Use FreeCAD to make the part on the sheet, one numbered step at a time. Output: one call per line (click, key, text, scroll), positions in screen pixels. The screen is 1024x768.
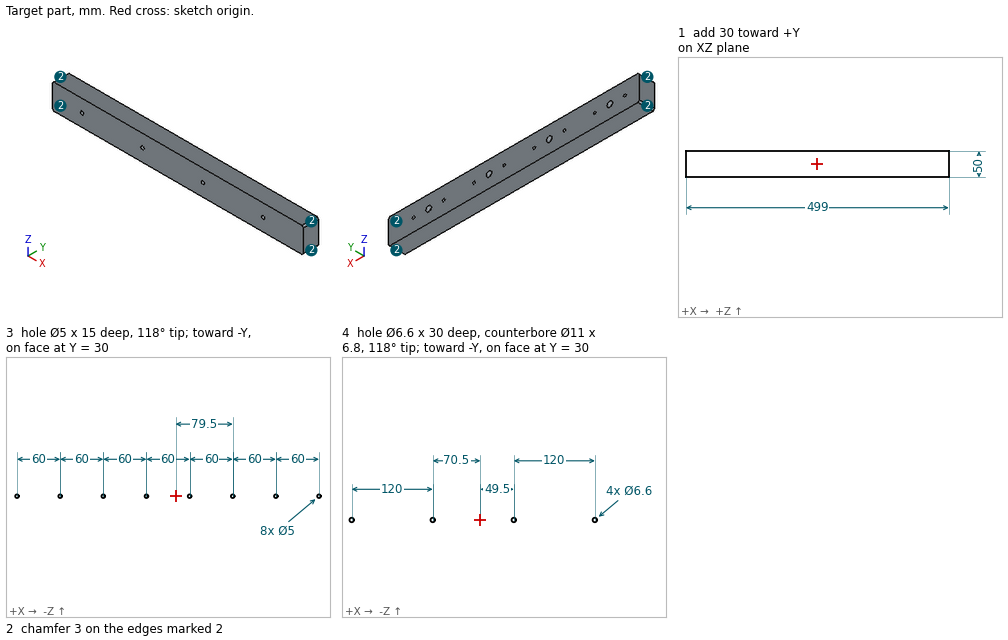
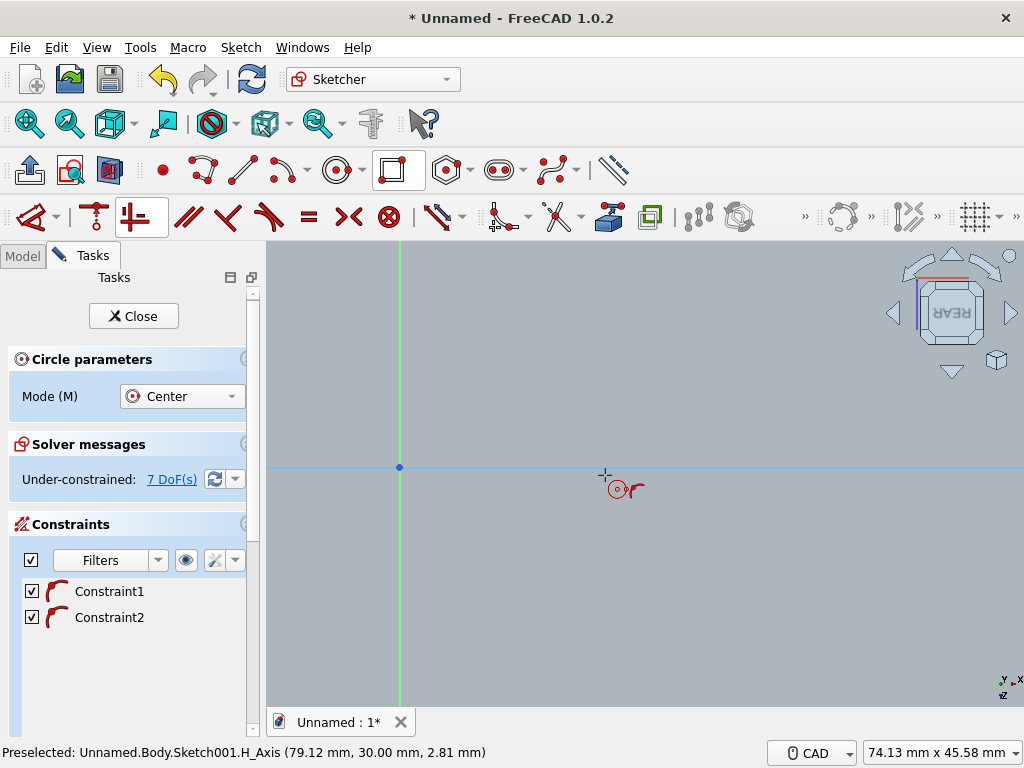
scroll(605, 475, down, 12)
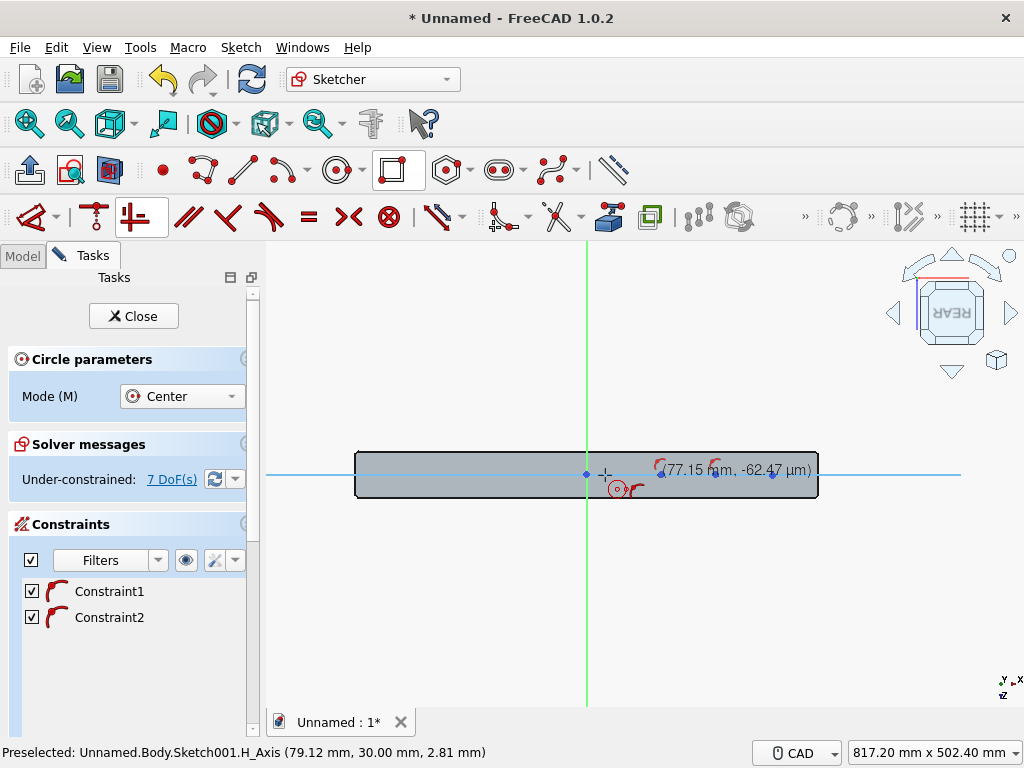
click(605, 475)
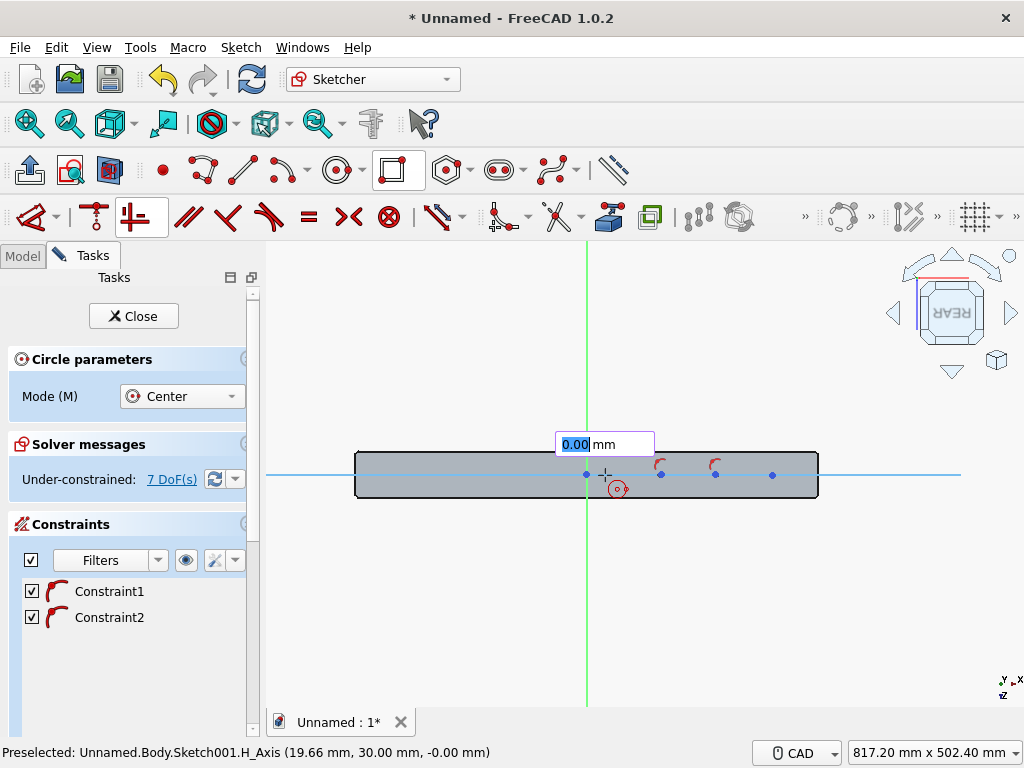
scroll(604, 477, up, 10)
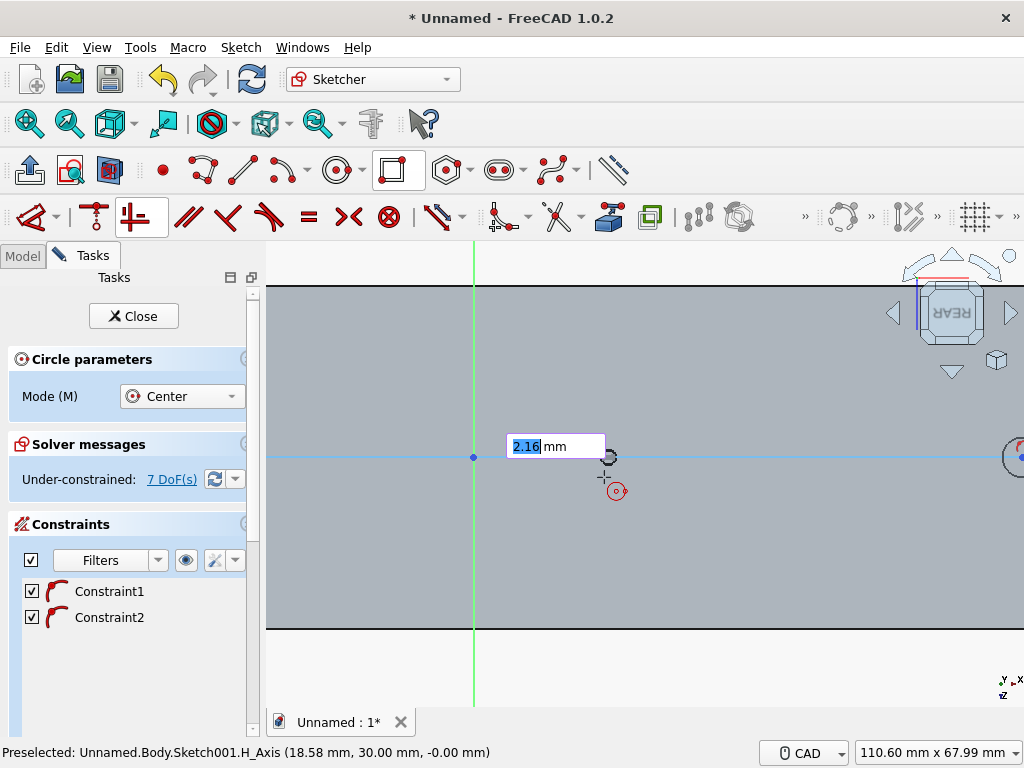
click(602, 474)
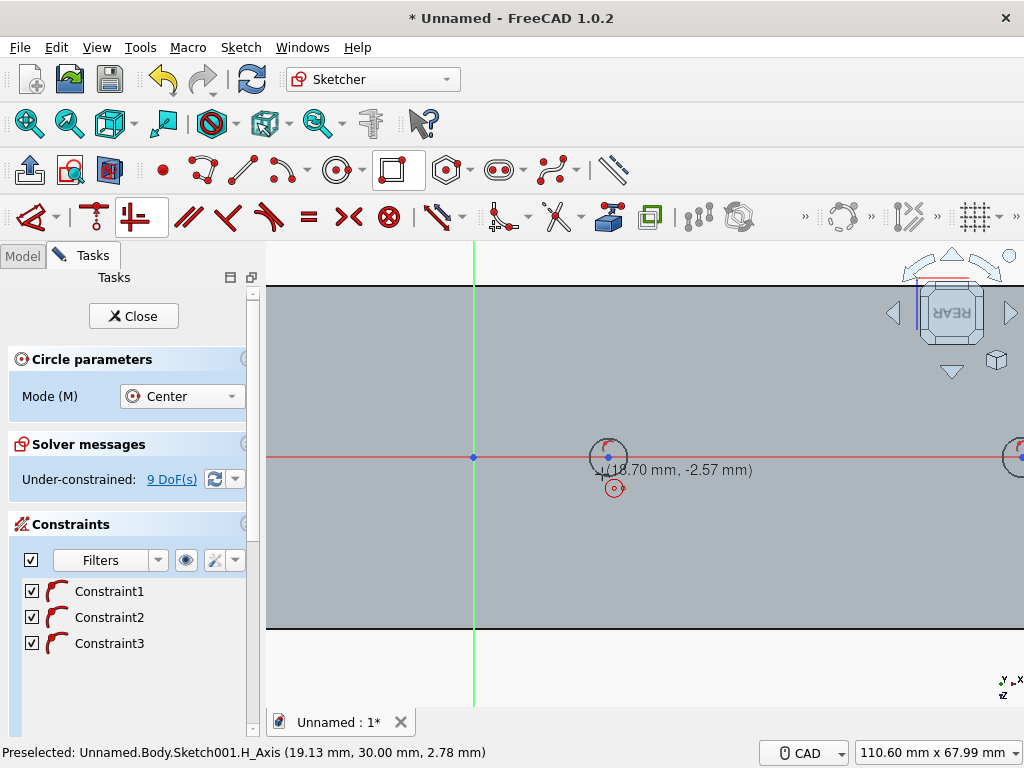
scroll(604, 477, down, 10)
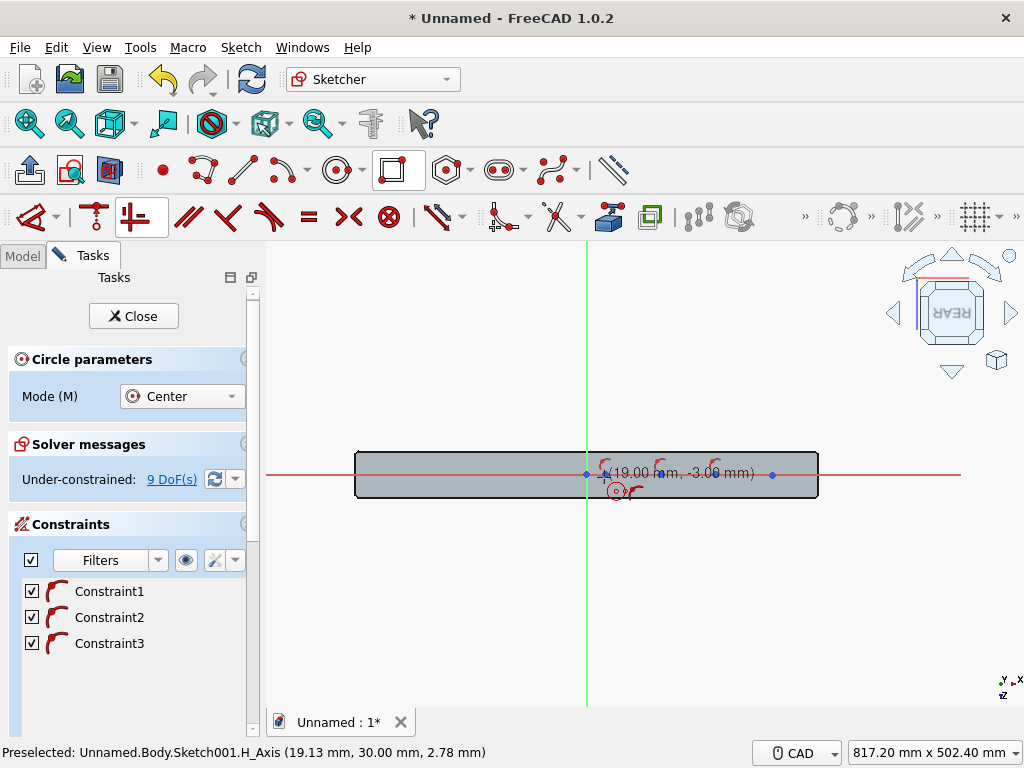
scroll(549, 475, up, 12)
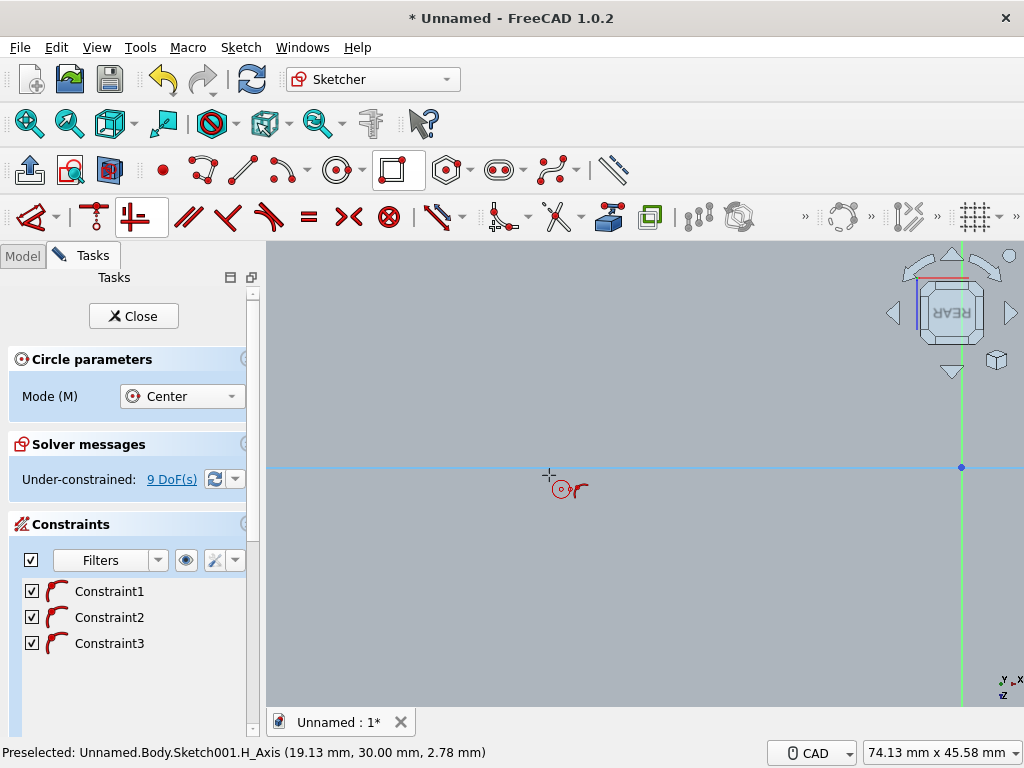
scroll(549, 475, down, 12)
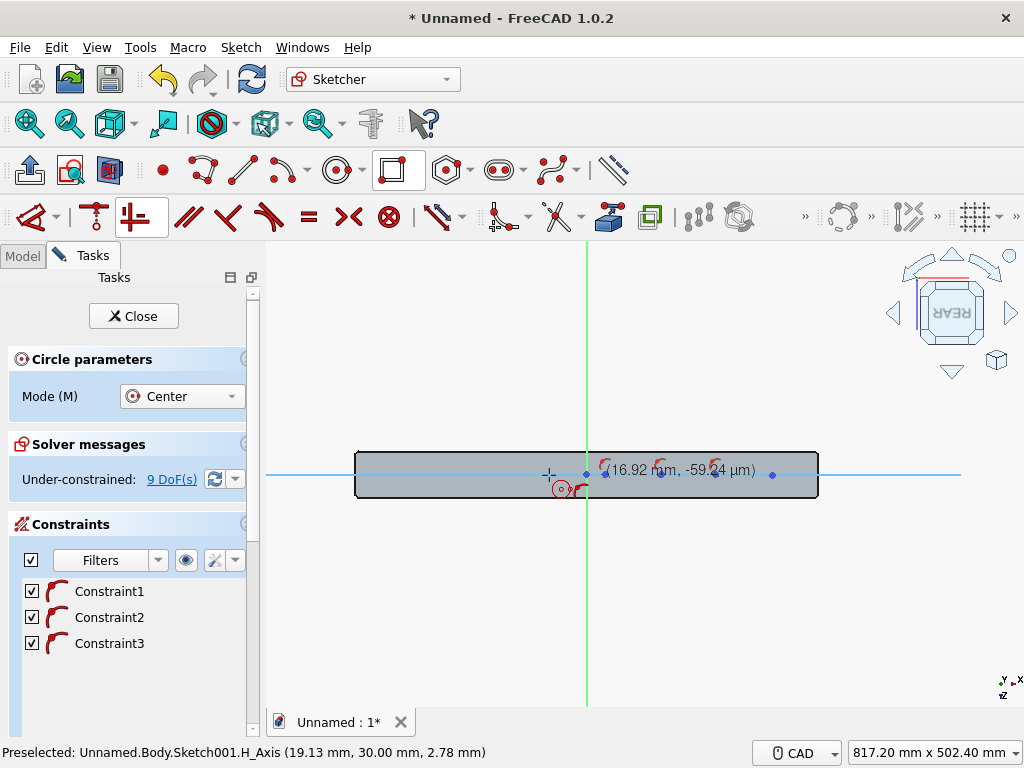
click(549, 475)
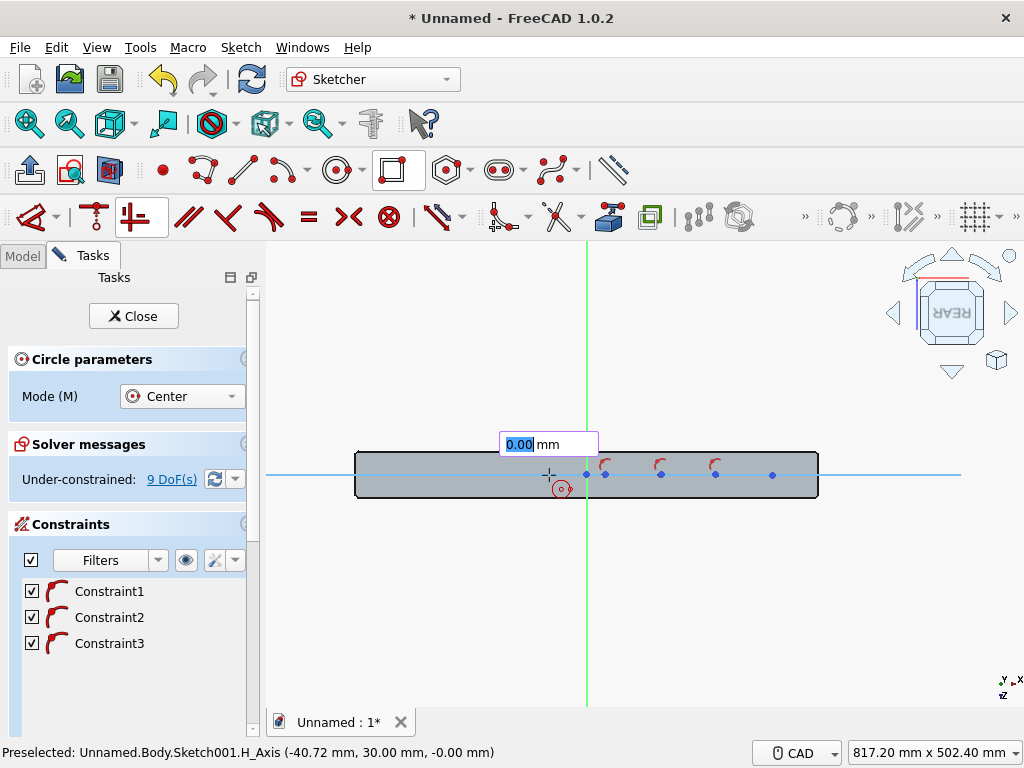
scroll(548, 477, up, 10)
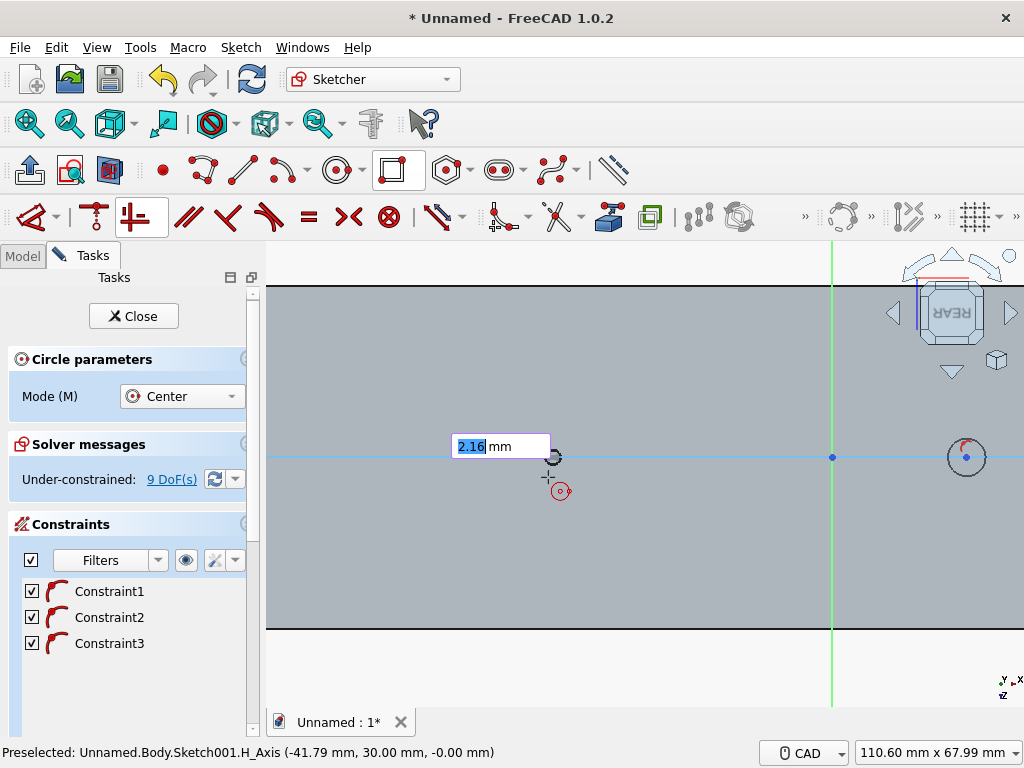
click(549, 474)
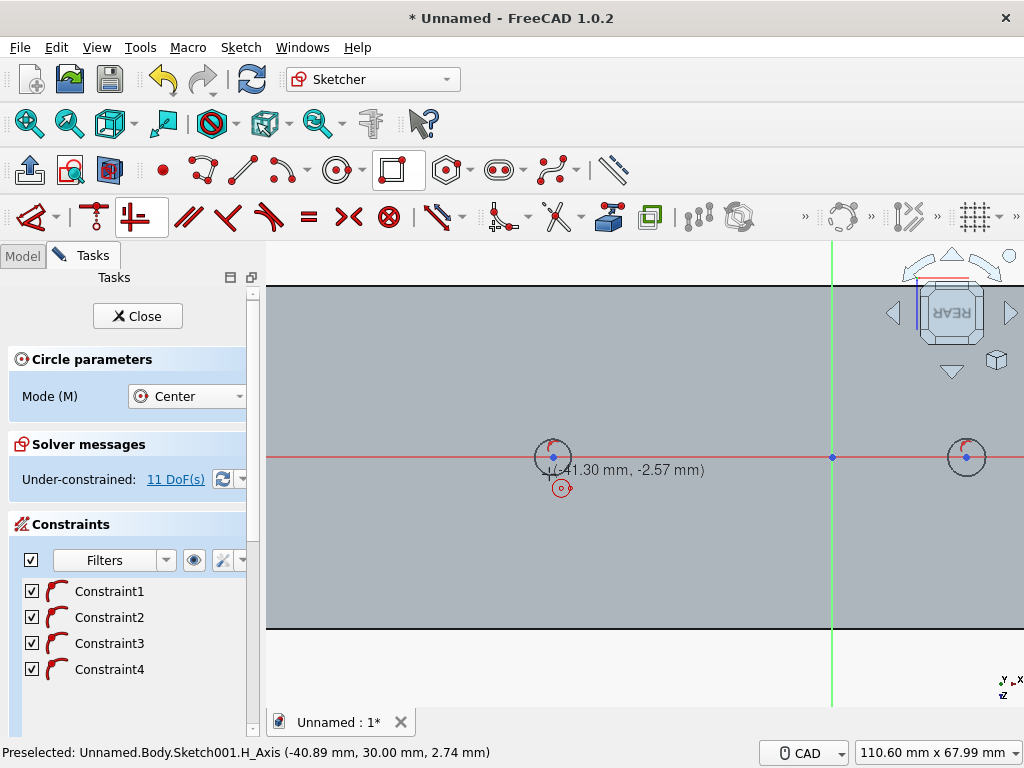
scroll(548, 477, down, 10)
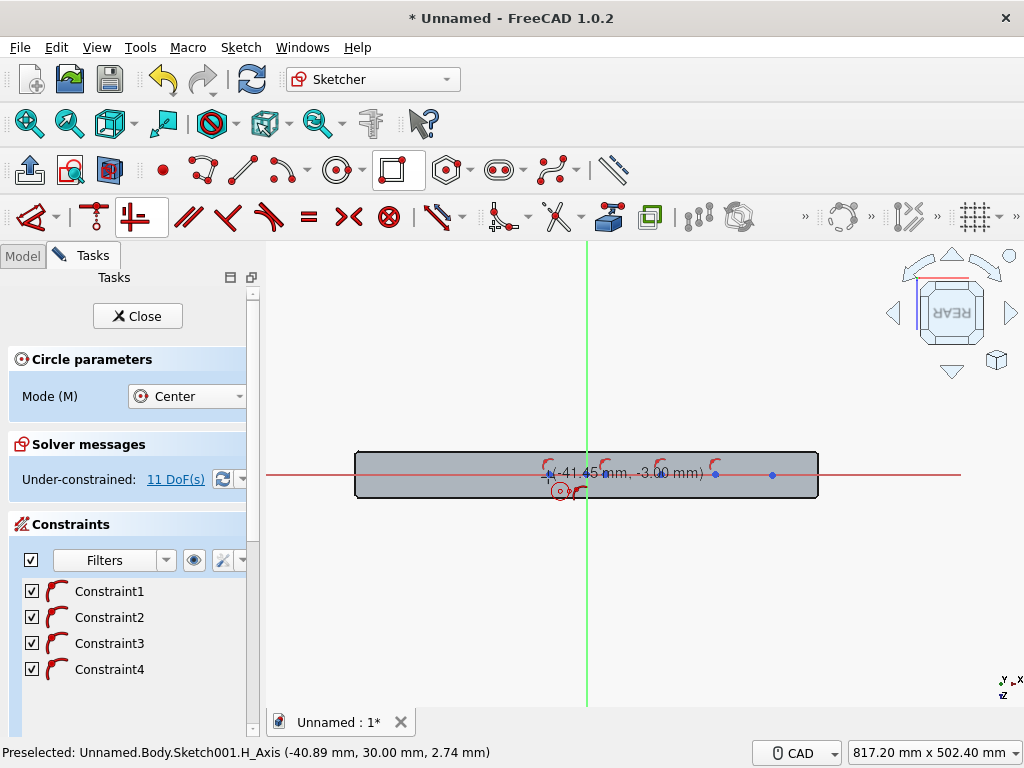
scroll(494, 475, up, 12)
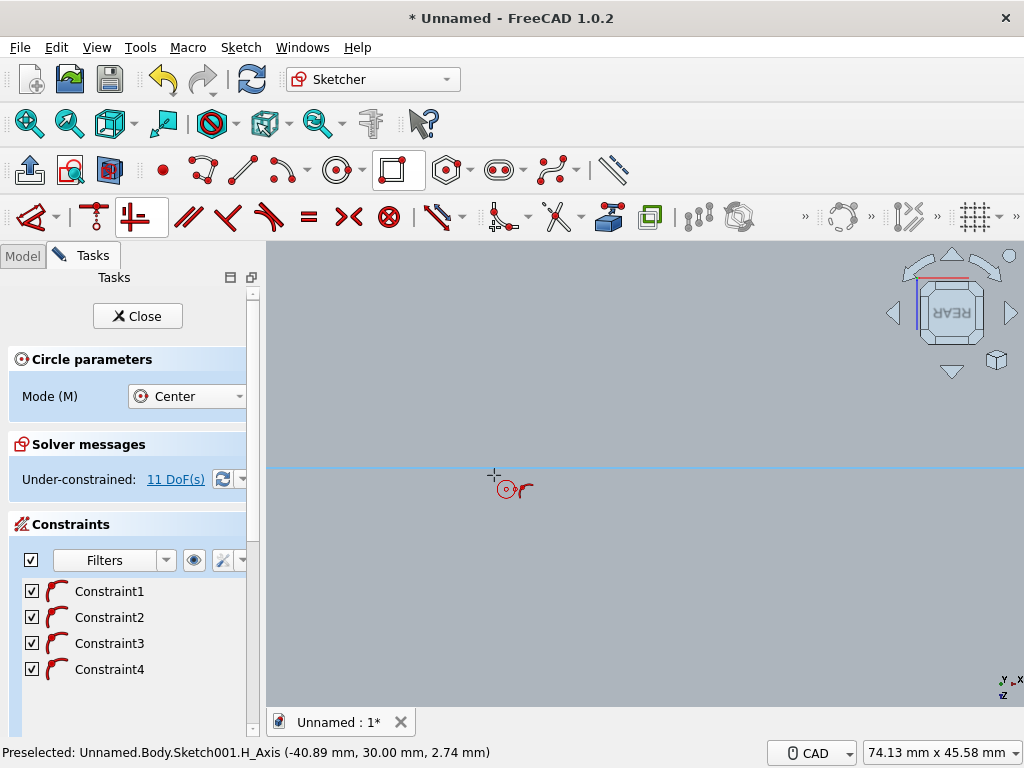
scroll(494, 475, down, 12)